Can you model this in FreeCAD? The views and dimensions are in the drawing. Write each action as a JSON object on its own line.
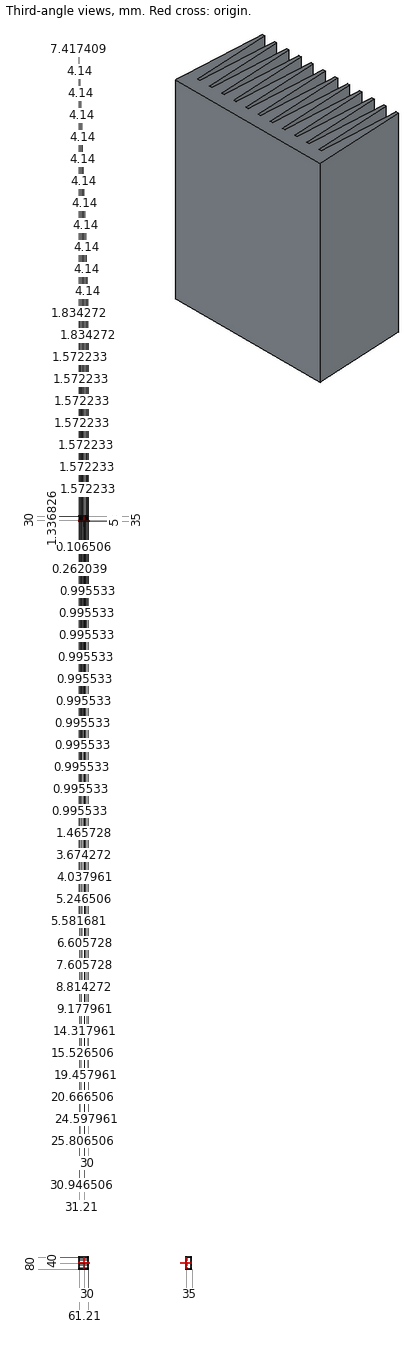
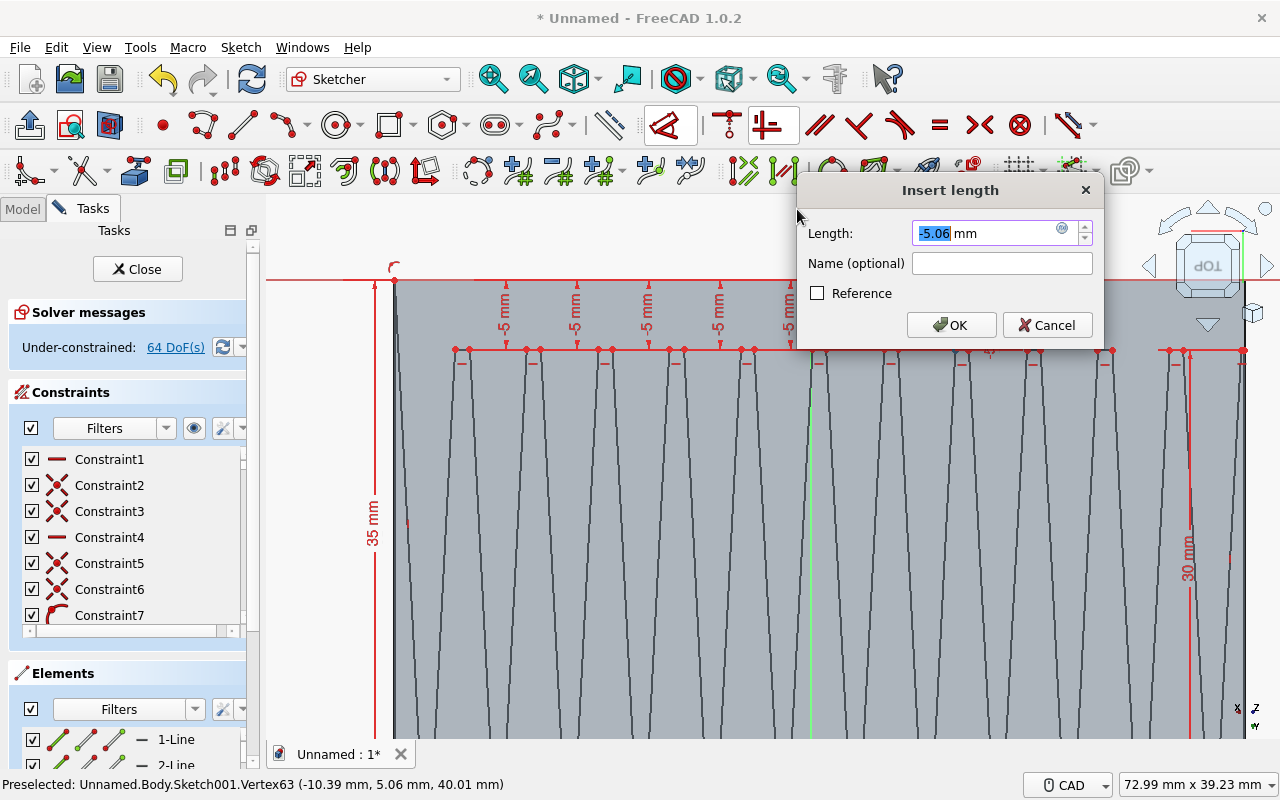
{"action": "type", "text": "-5"}
{"action": "key", "text": "Return"}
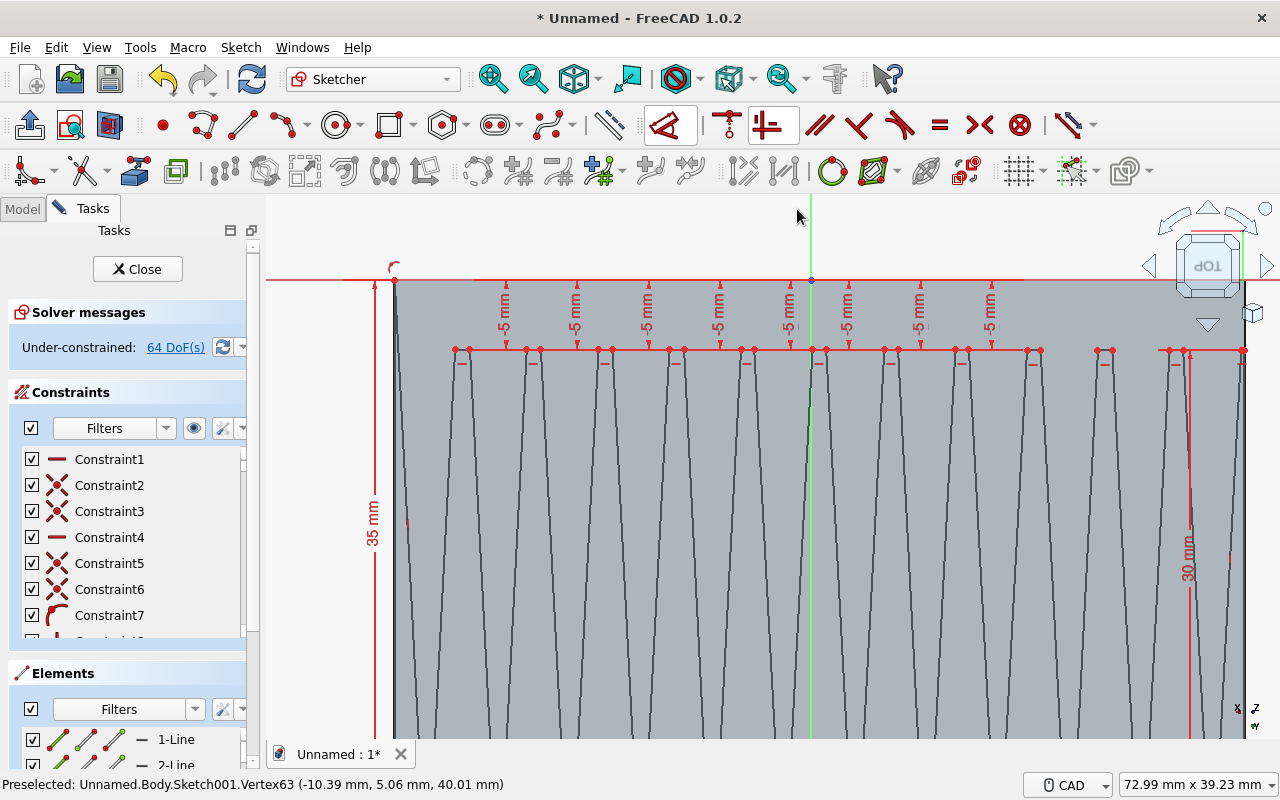
{"action": "left_click", "coordinate": [1027, 350]}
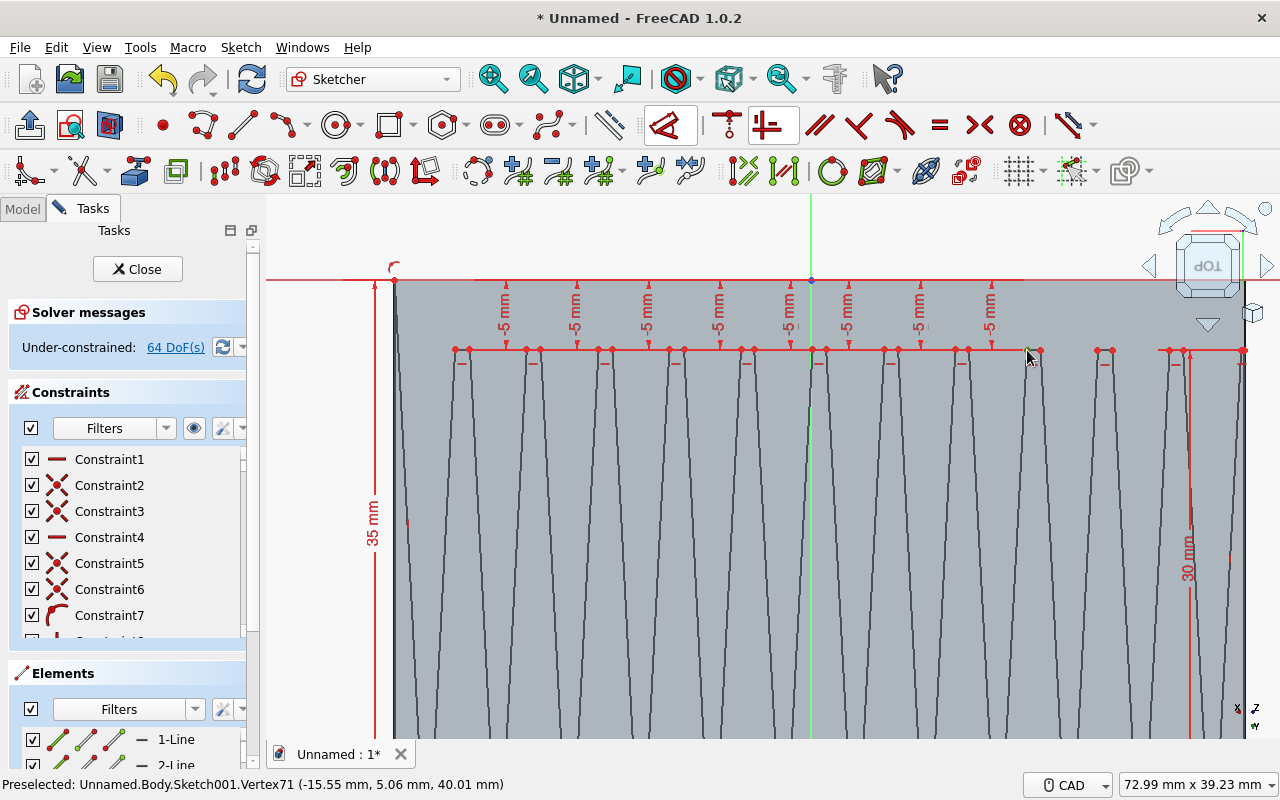
{"action": "left_click", "coordinate": [692, 126]}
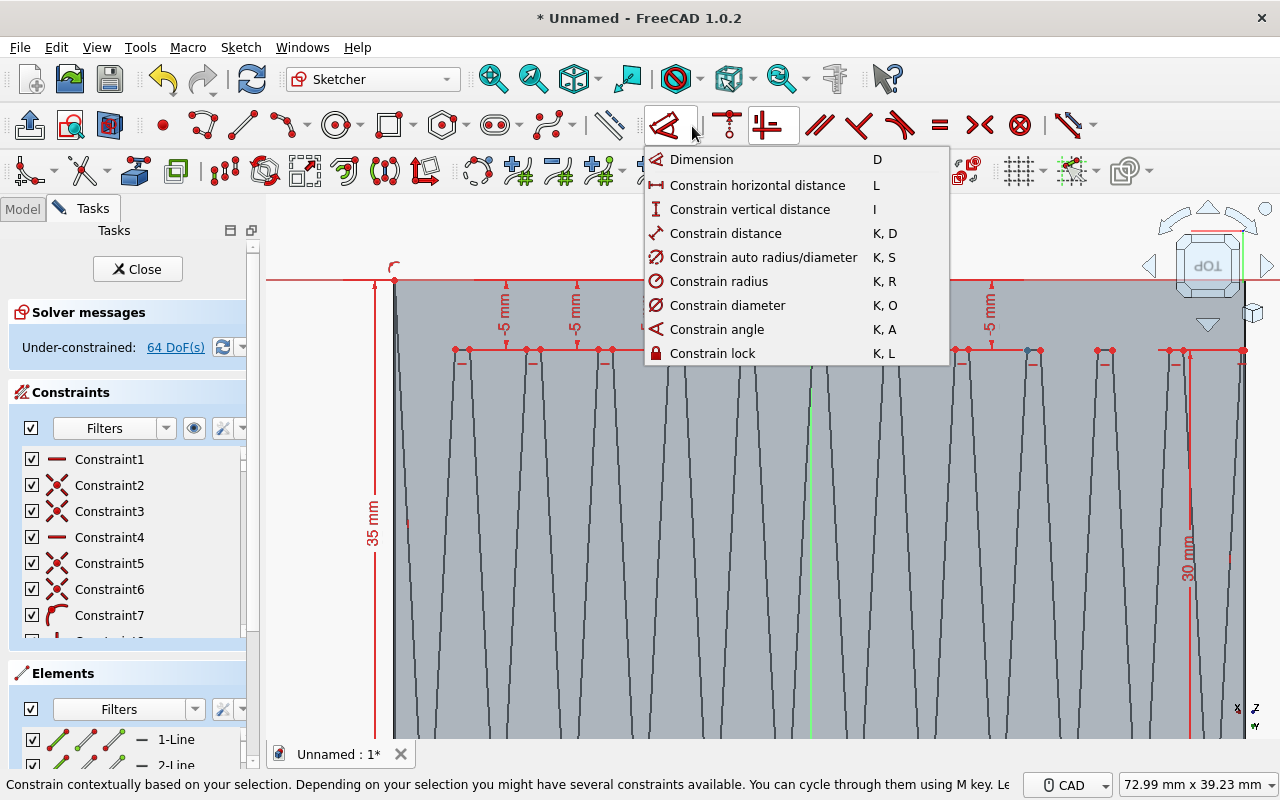
{"action": "left_click", "coordinate": [797, 209]}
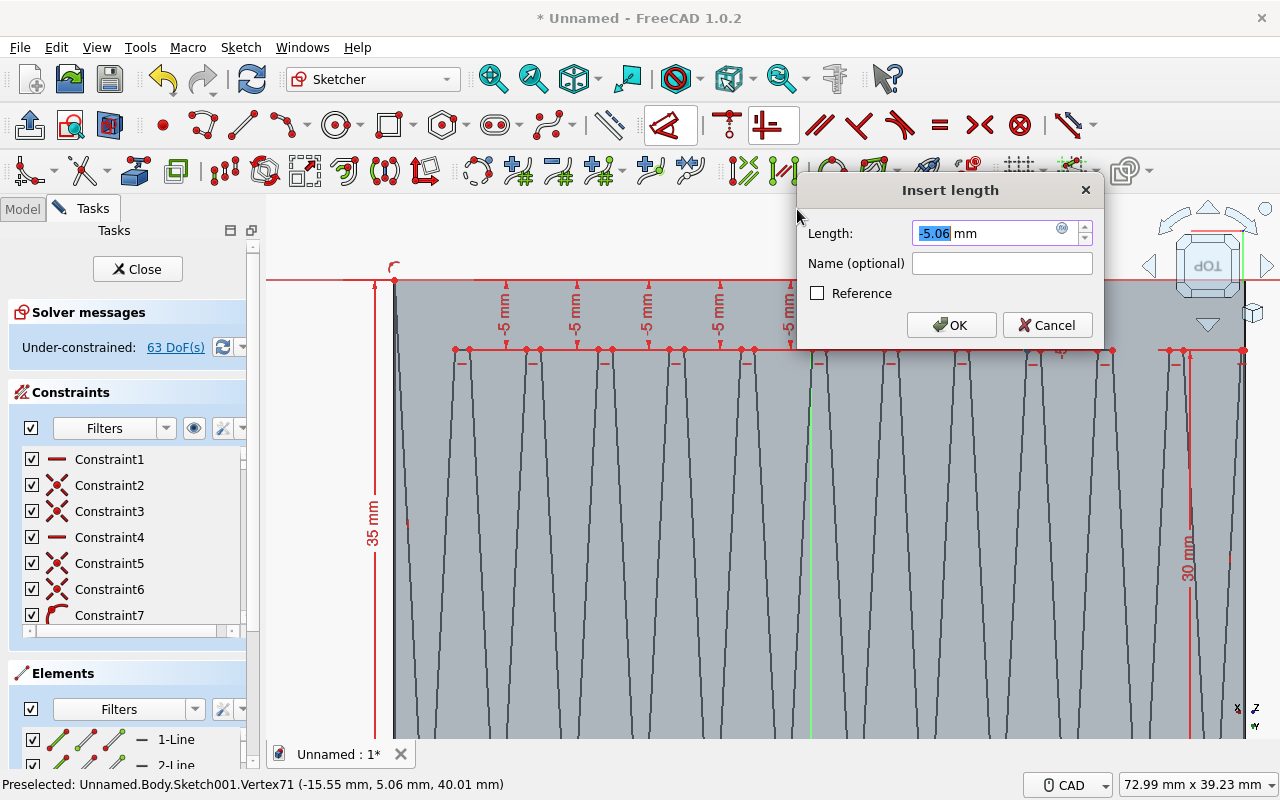
{"action": "type", "text": "-5"}
{"action": "key", "text": "Return"}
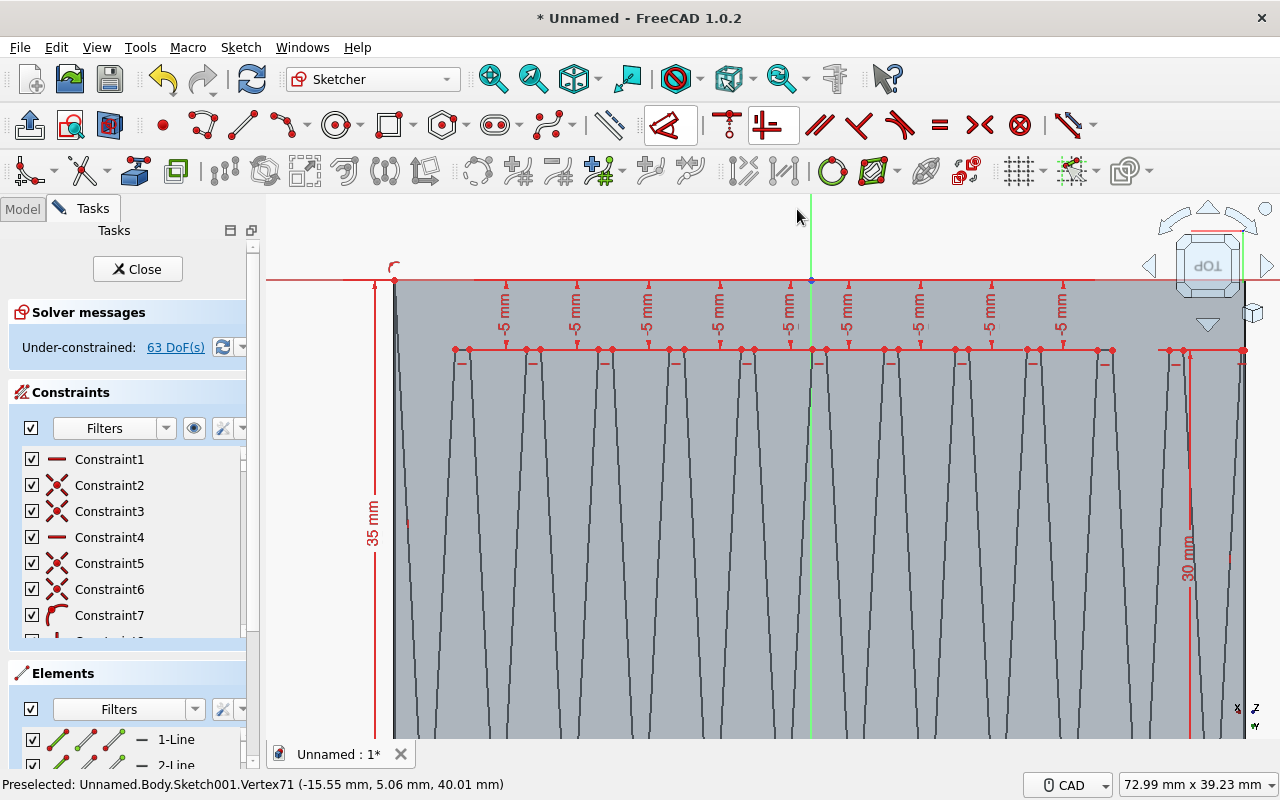
{"action": "left_click", "coordinate": [1098, 350]}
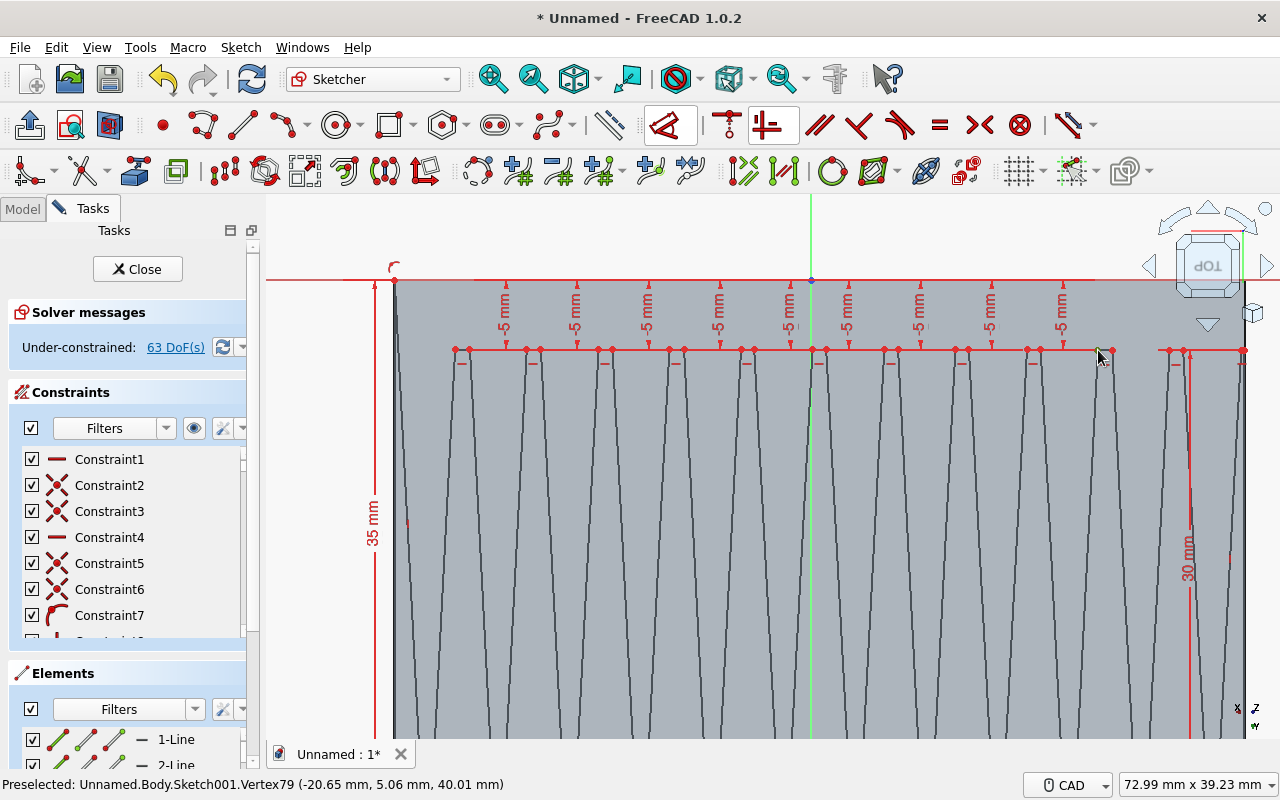
{"action": "left_click", "coordinate": [692, 126]}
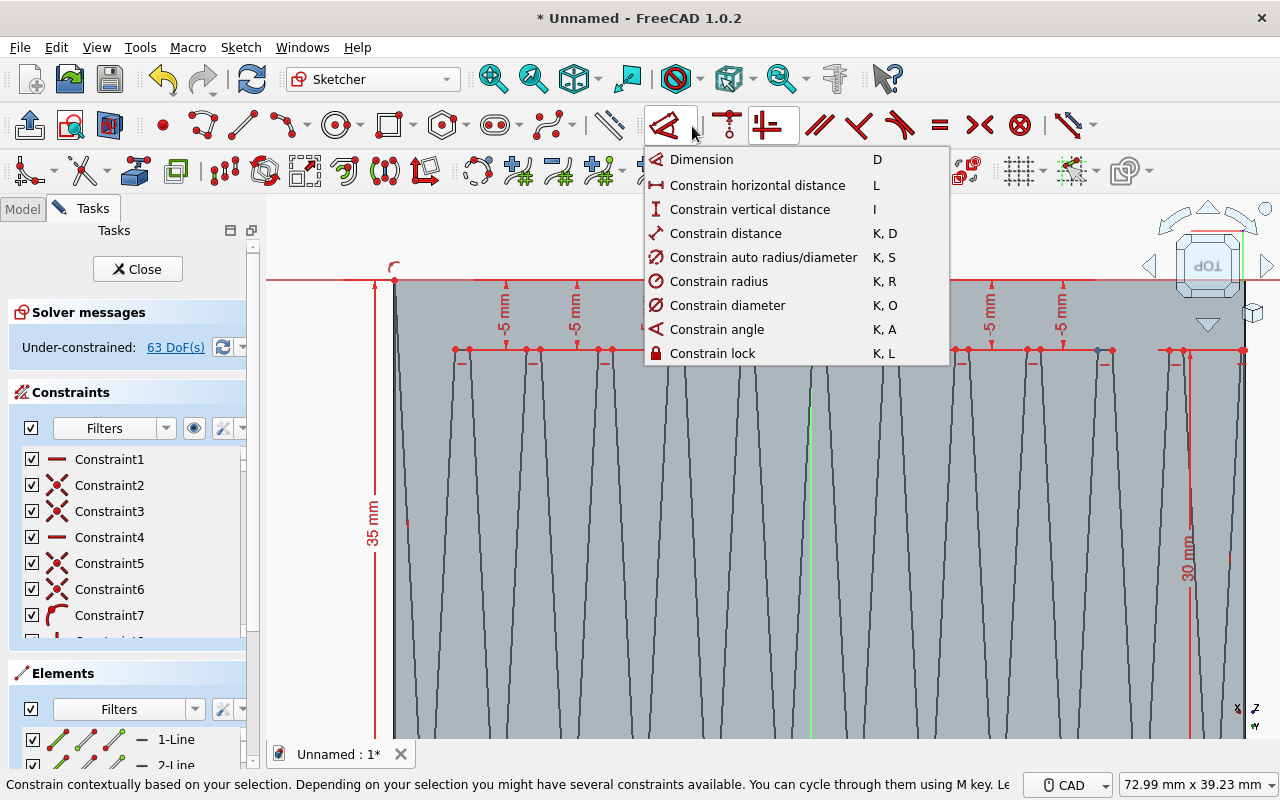
{"action": "left_click", "coordinate": [797, 209]}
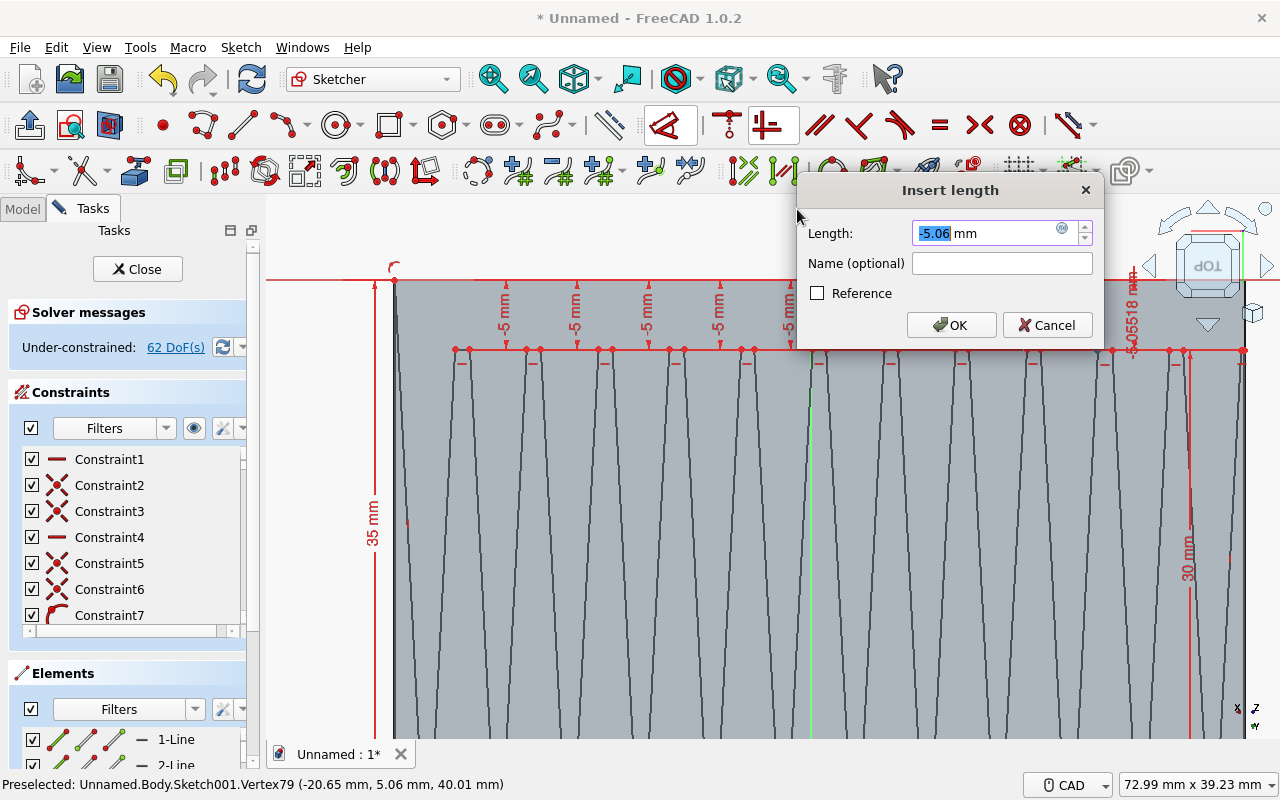
{"action": "type", "text": "-5"}
{"action": "key", "text": "Return"}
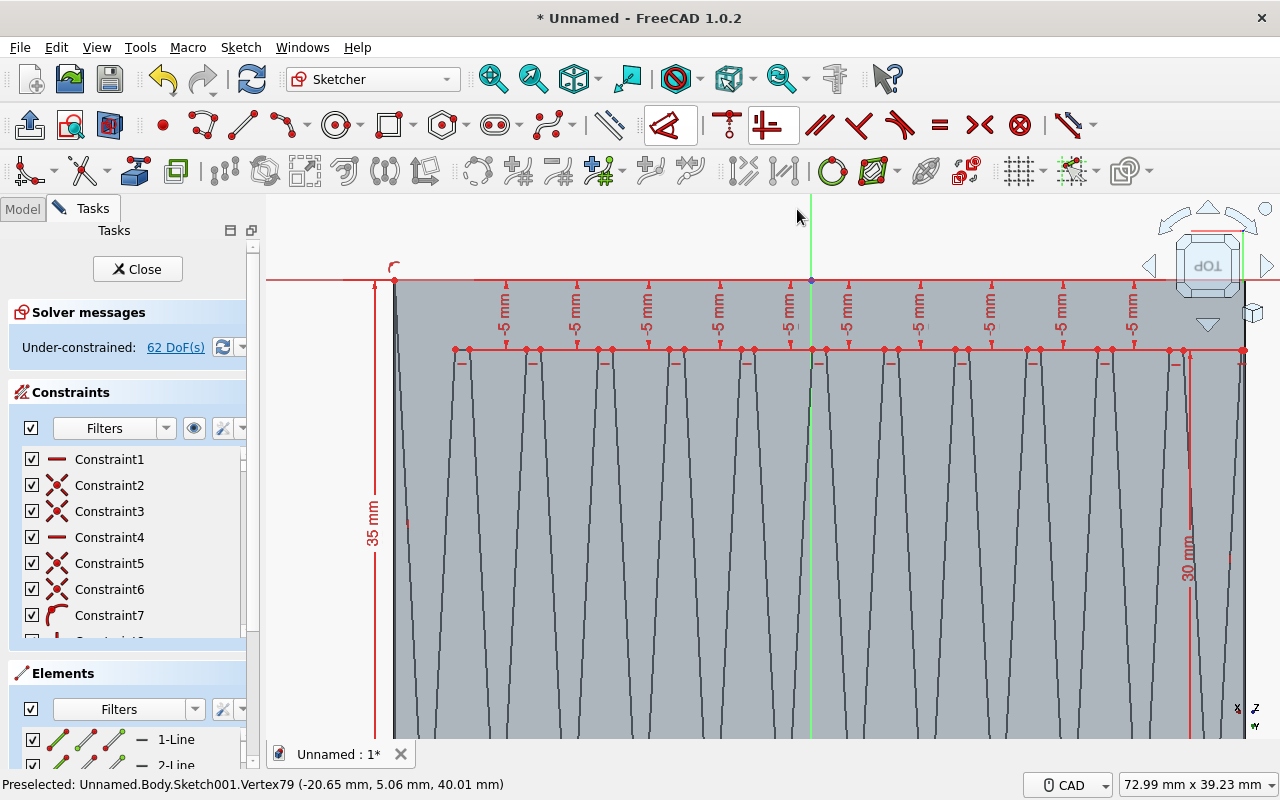
{"action": "scroll", "coordinate": [471, 351], "scroll_direction": "down", "scroll_amount": 2}